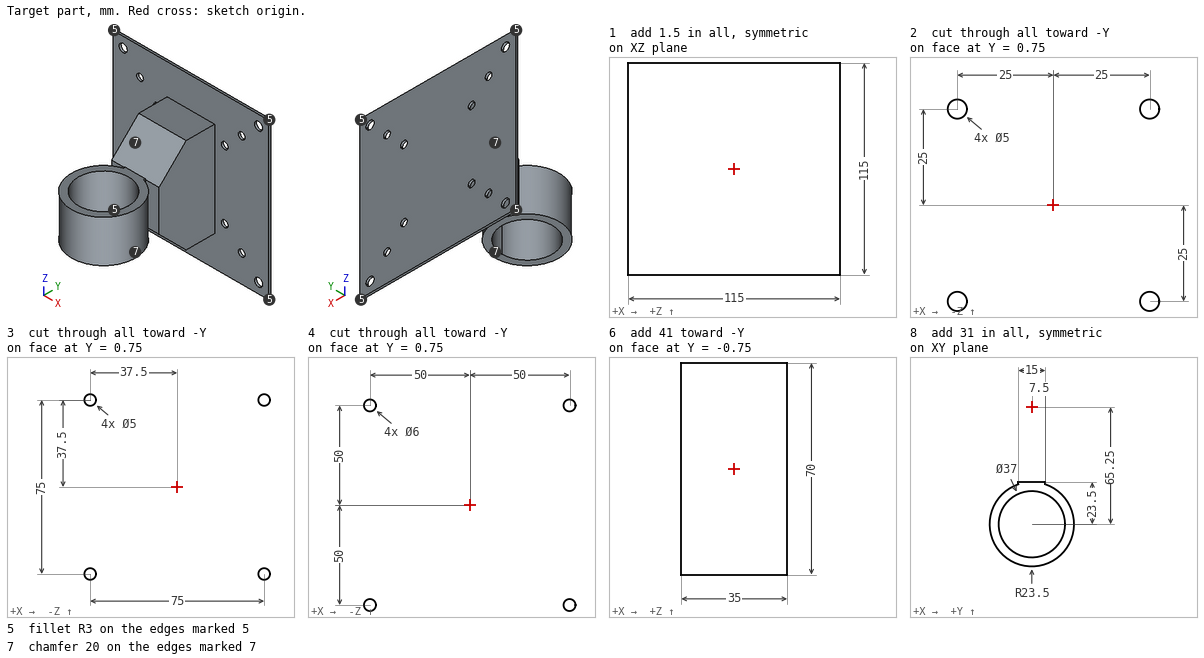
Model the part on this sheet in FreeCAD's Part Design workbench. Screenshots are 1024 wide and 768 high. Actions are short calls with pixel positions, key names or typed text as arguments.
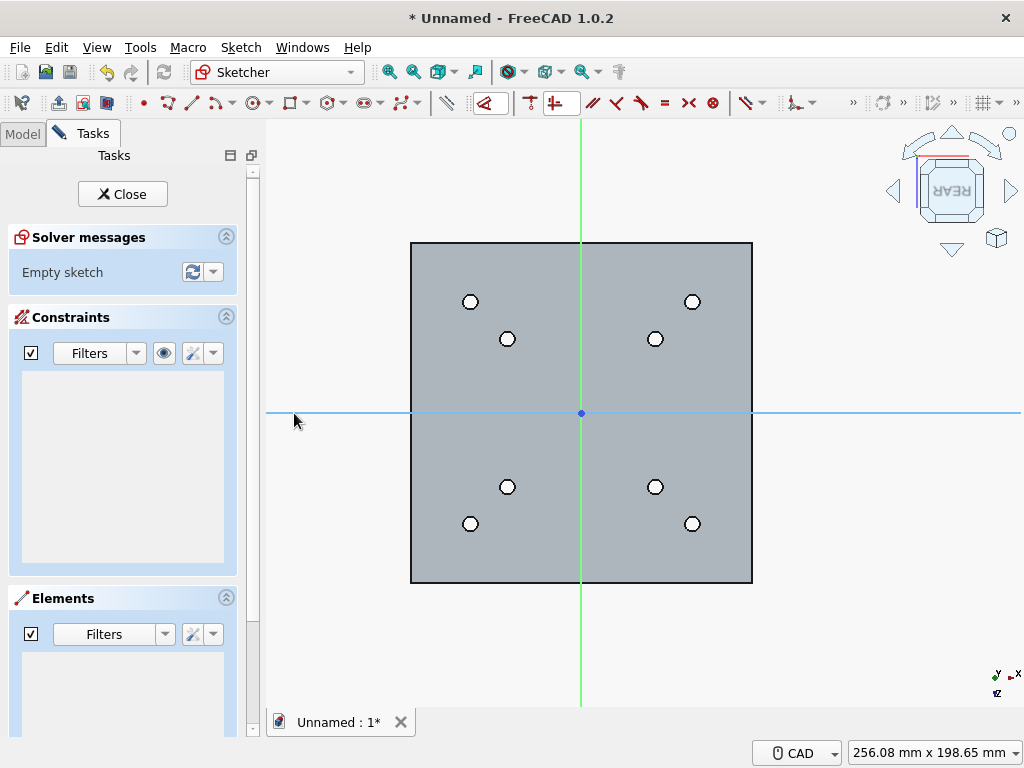
key(g)
key(c)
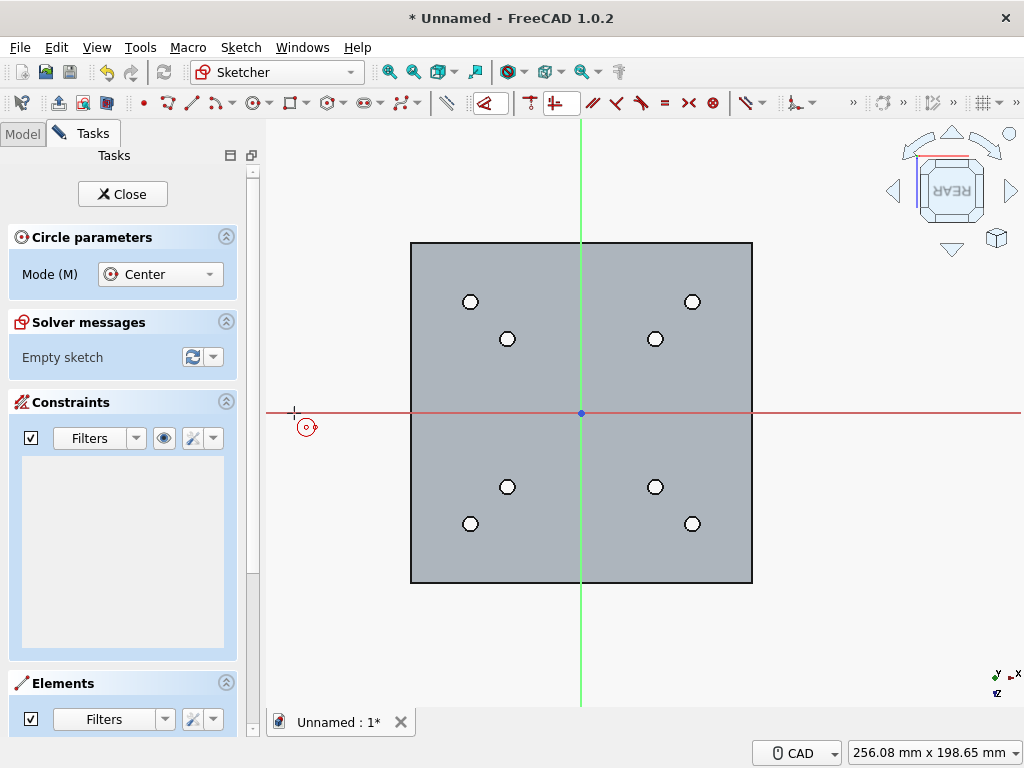
scroll(433, 265, up, 5)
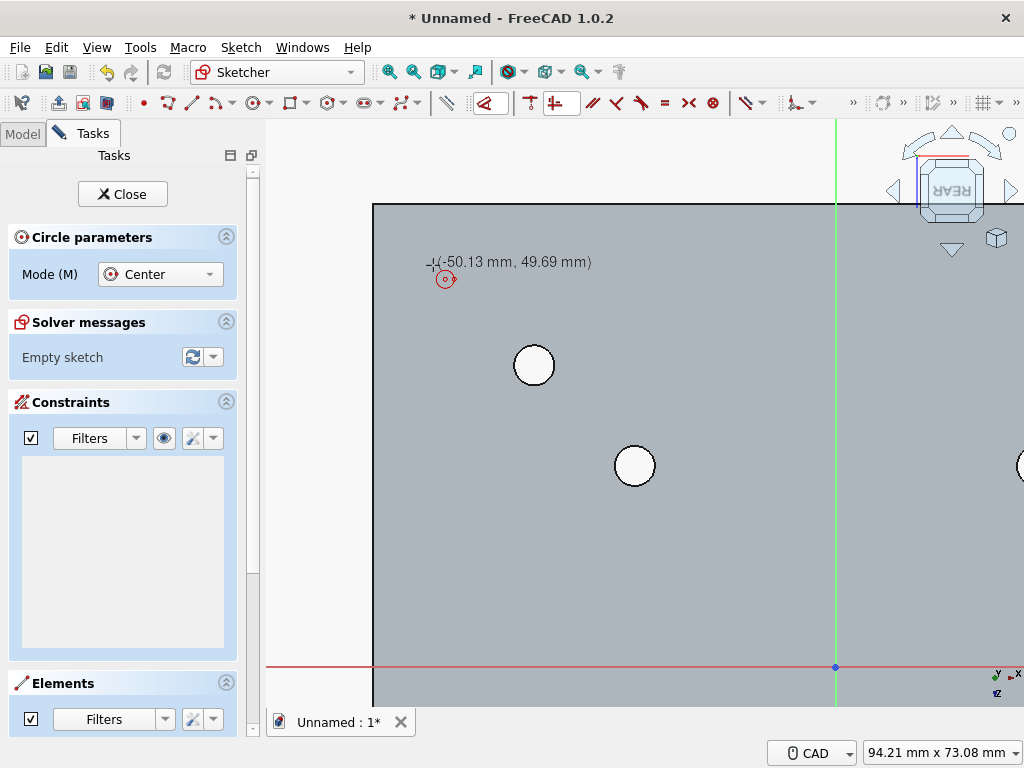
click(434, 265)
click(451, 248)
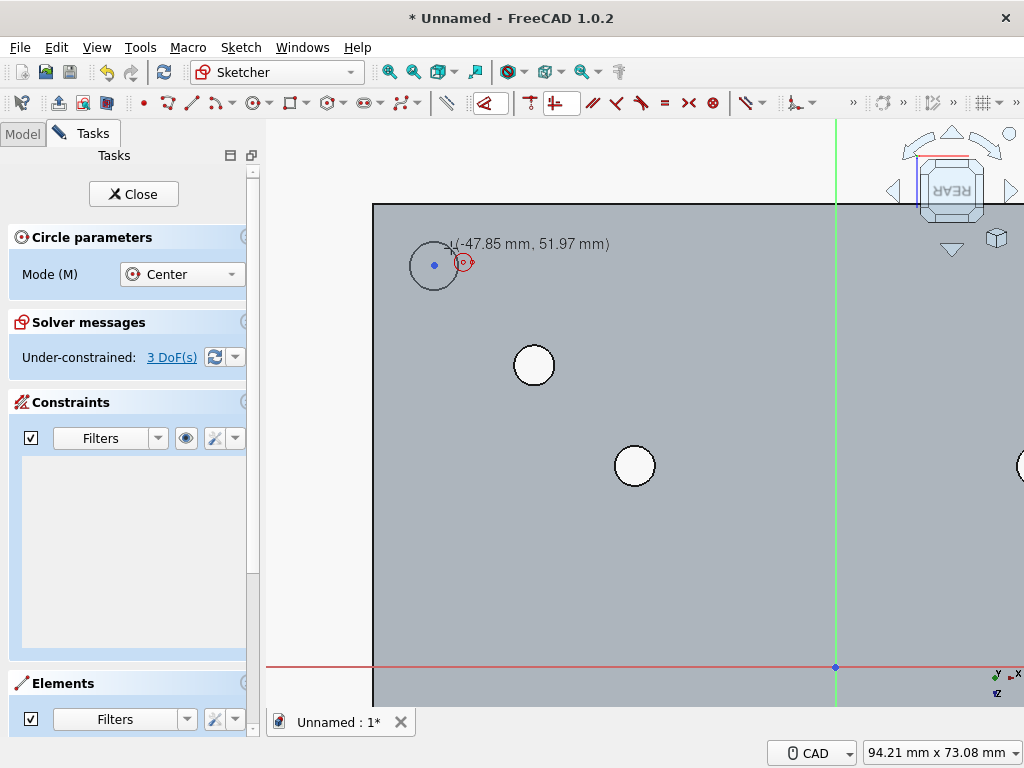
scroll(365, 206, down, 4)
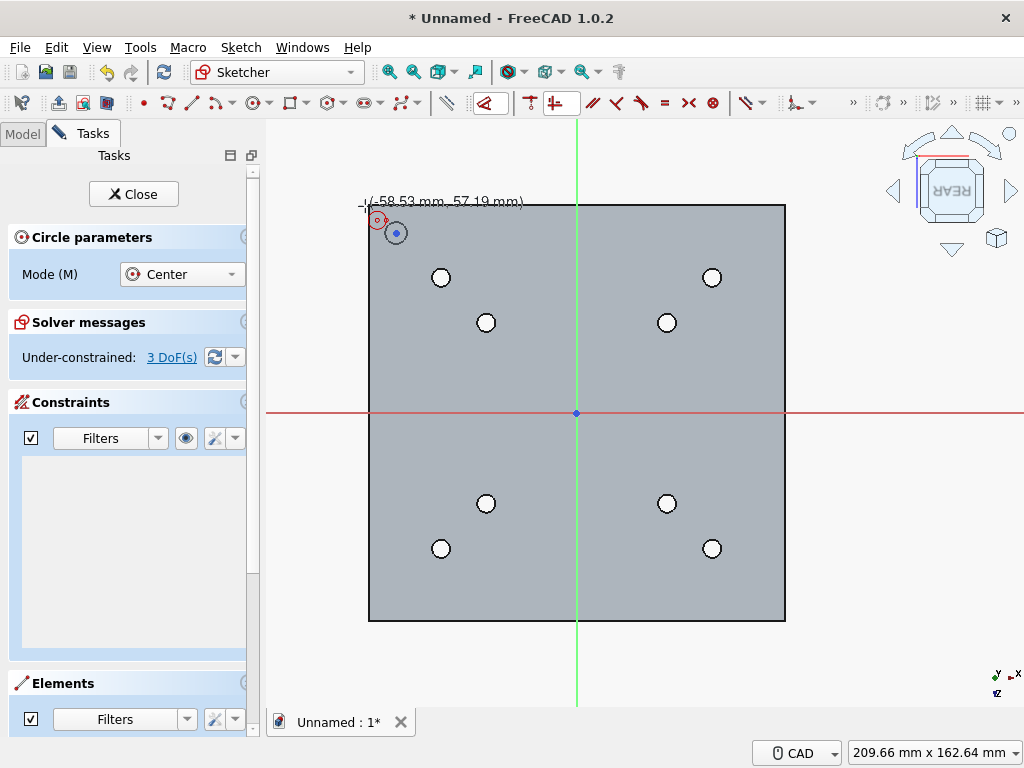
scroll(757, 233, up, 4)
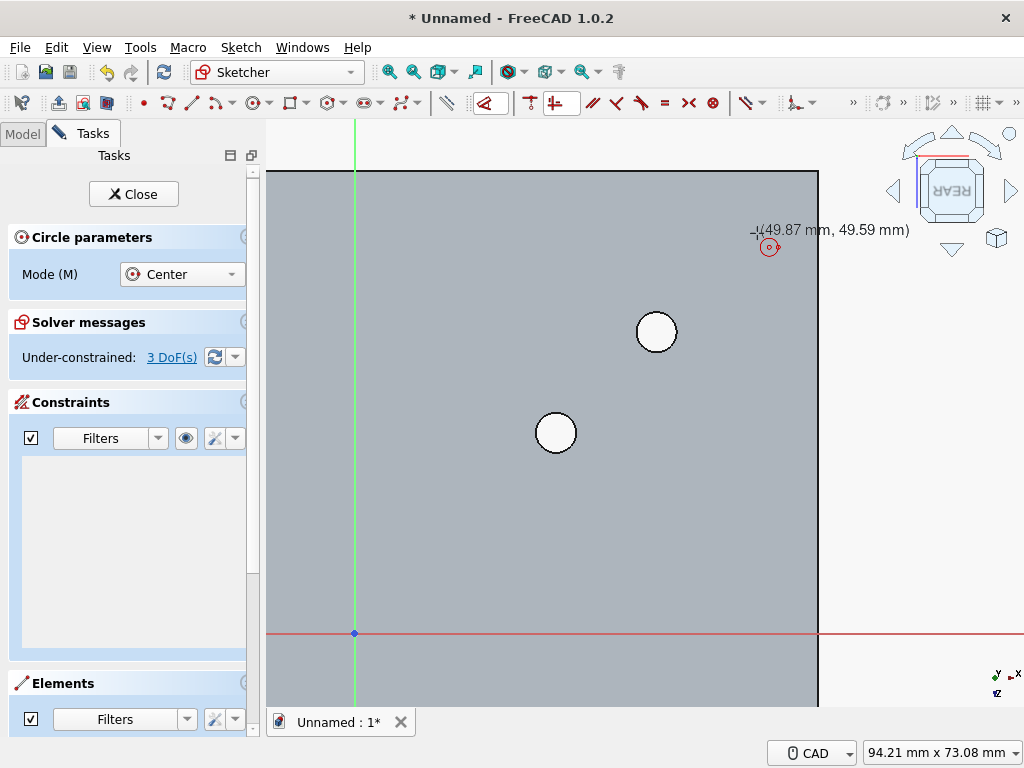
click(757, 232)
click(774, 215)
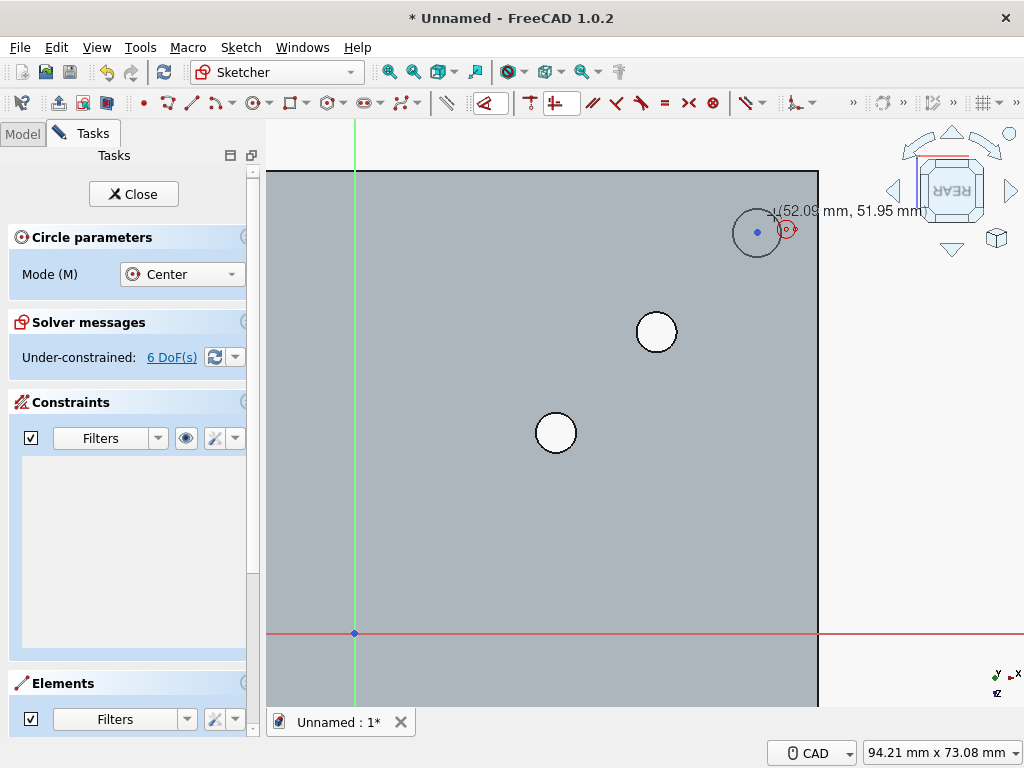
scroll(757, 233, down, 4)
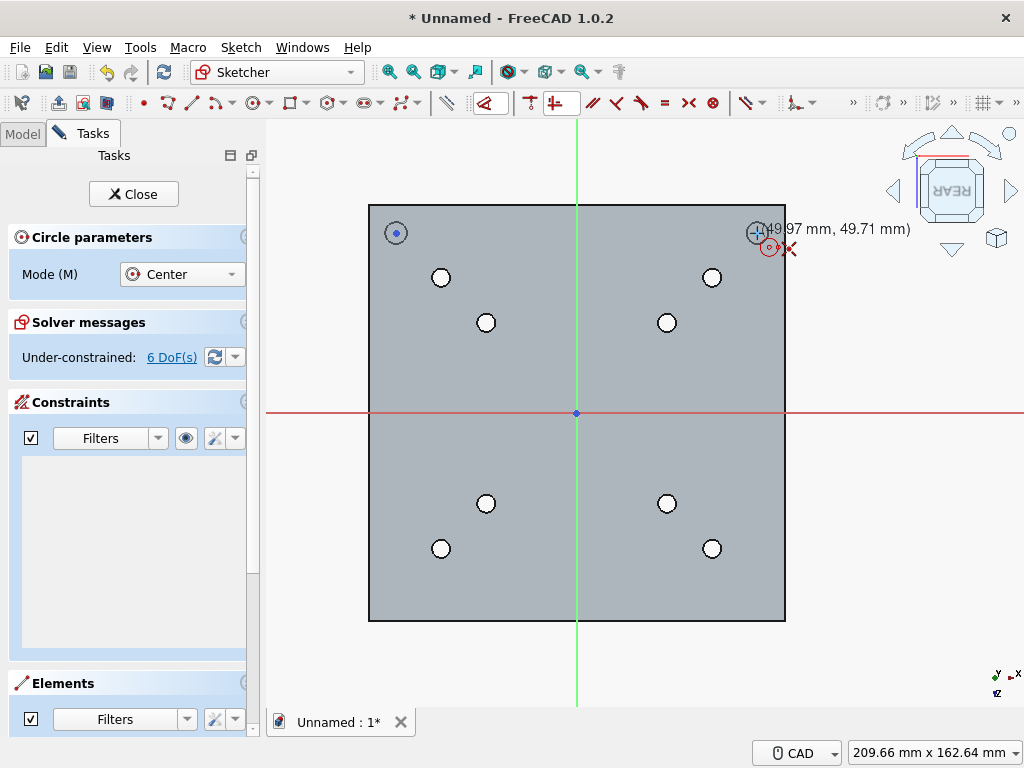
scroll(396, 594, up, 4)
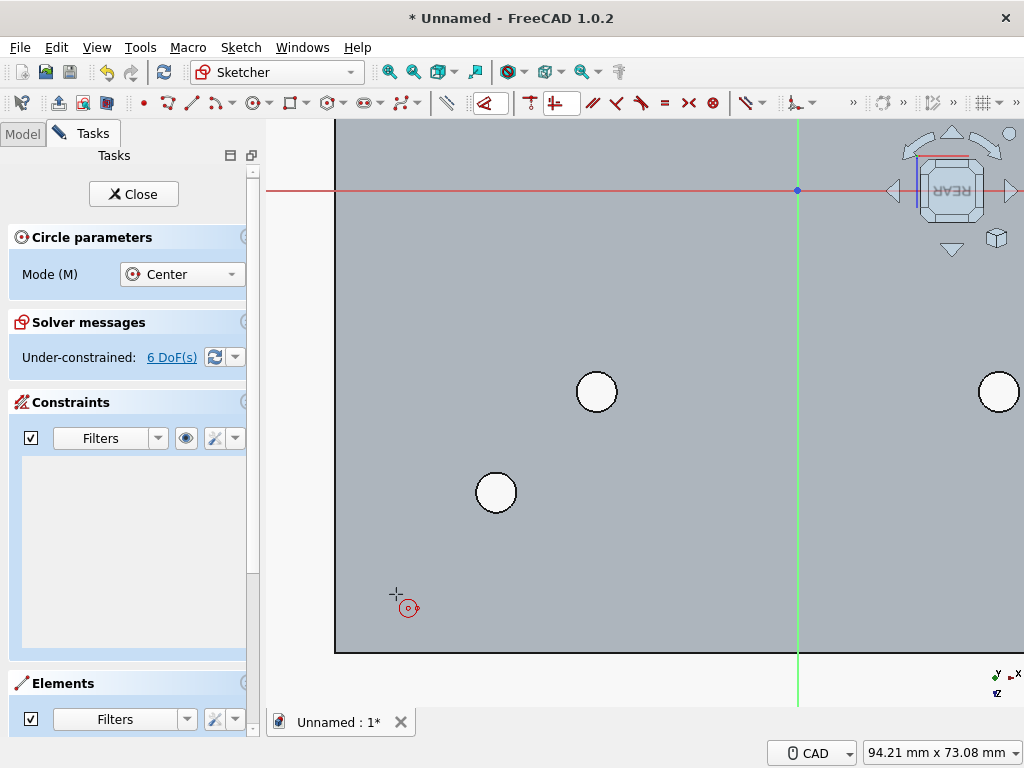
click(396, 593)
click(413, 576)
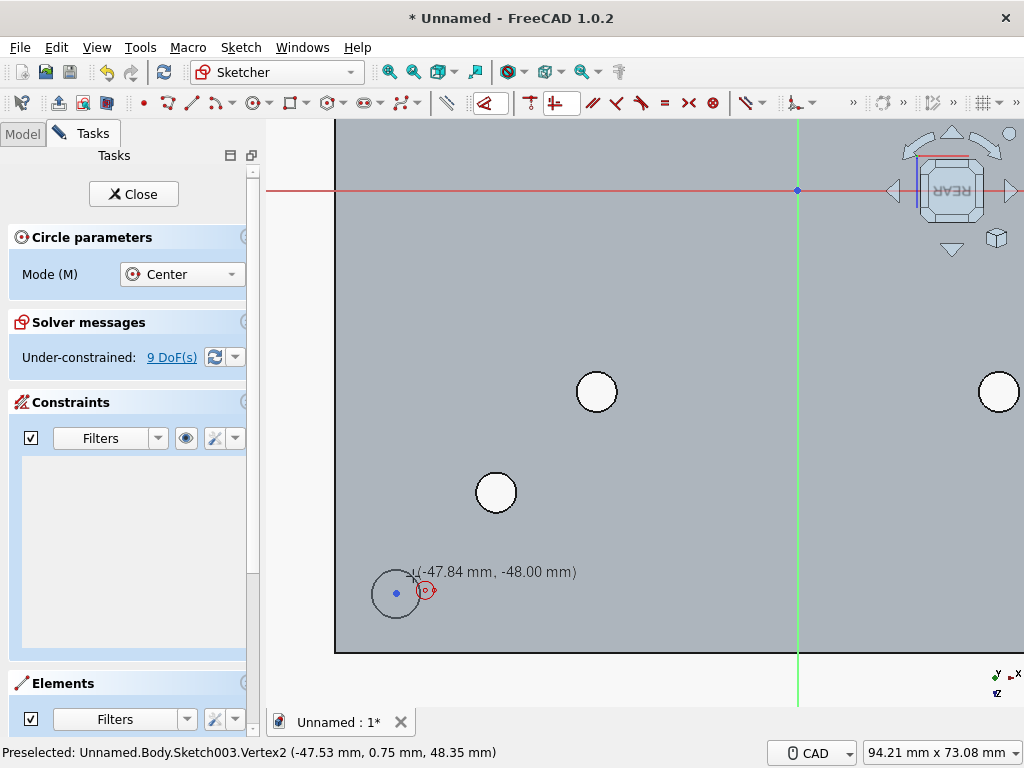
scroll(396, 594, down, 4)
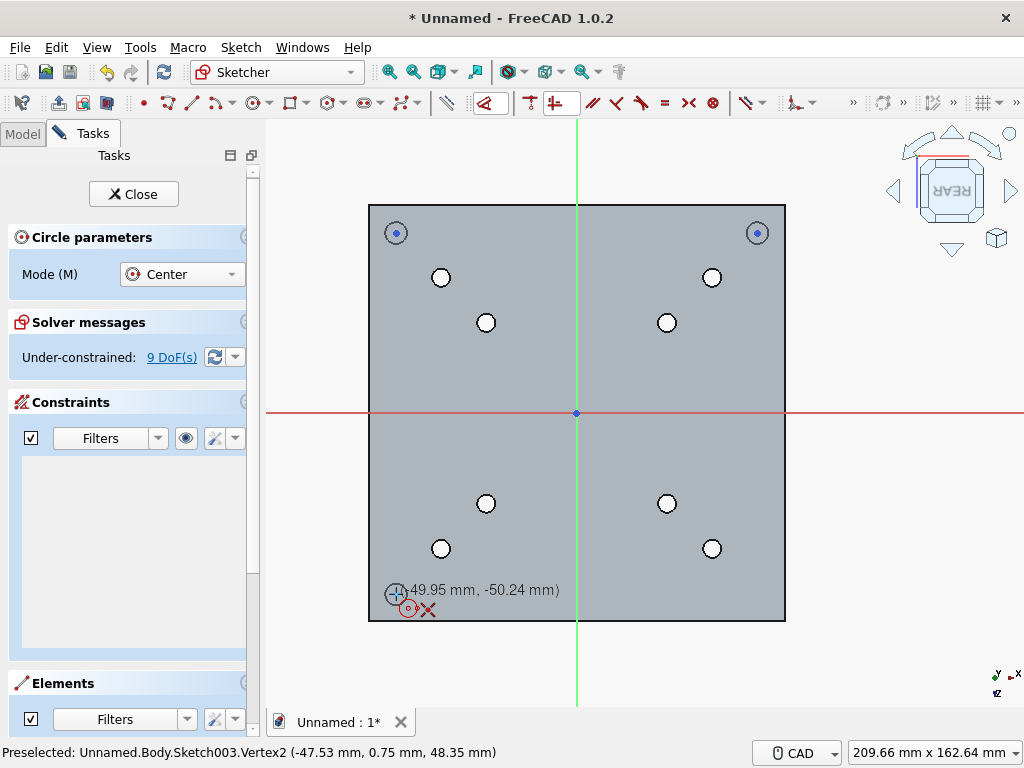
scroll(757, 594, up, 4)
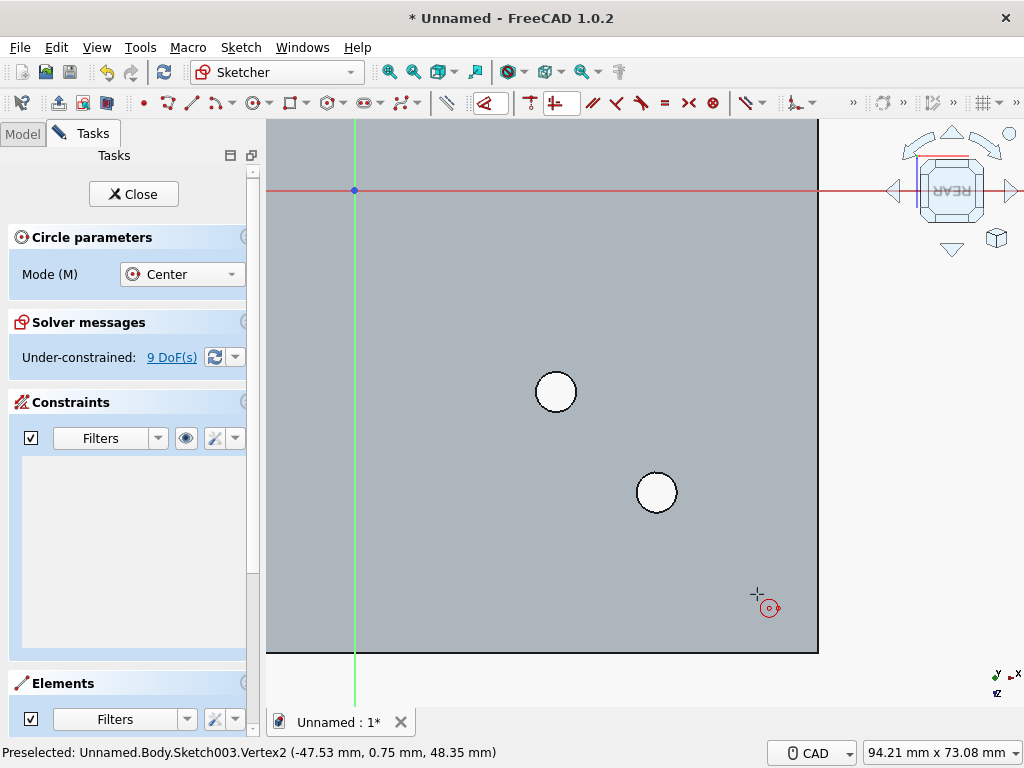
click(757, 593)
click(774, 576)
key(Escape)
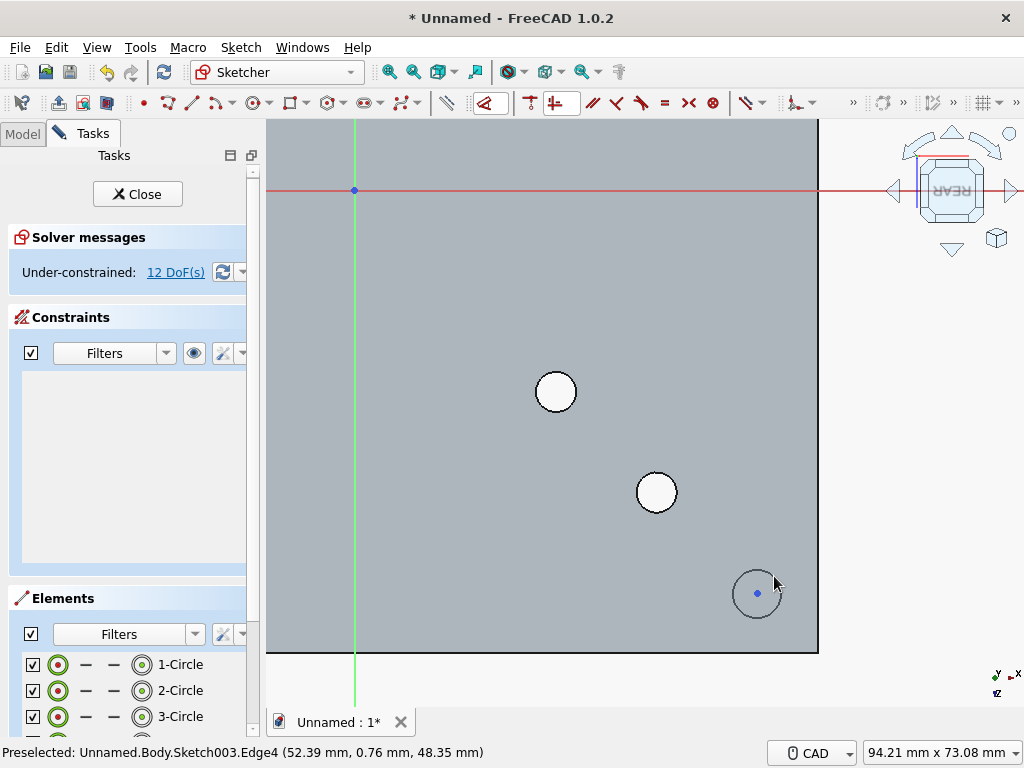
scroll(757, 594, down, 4)